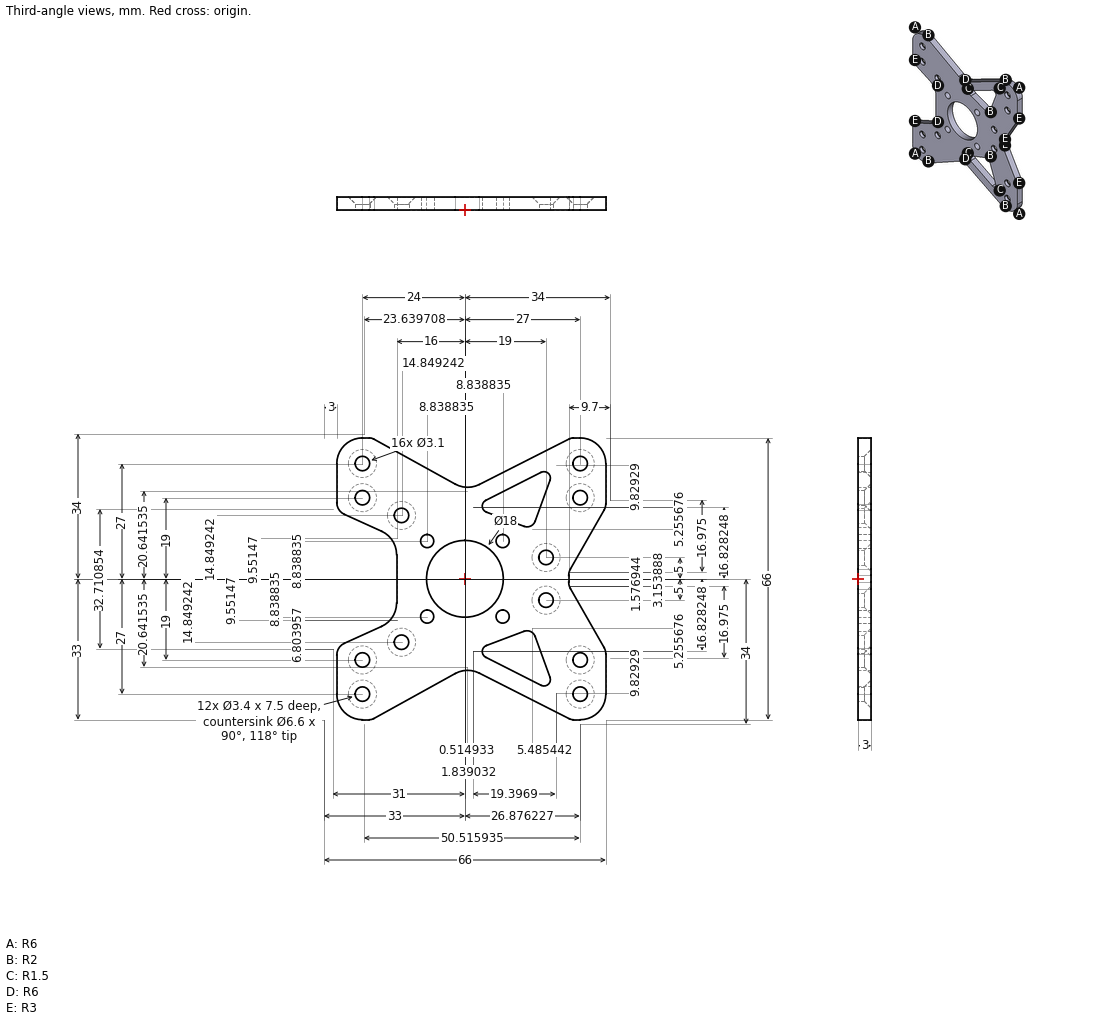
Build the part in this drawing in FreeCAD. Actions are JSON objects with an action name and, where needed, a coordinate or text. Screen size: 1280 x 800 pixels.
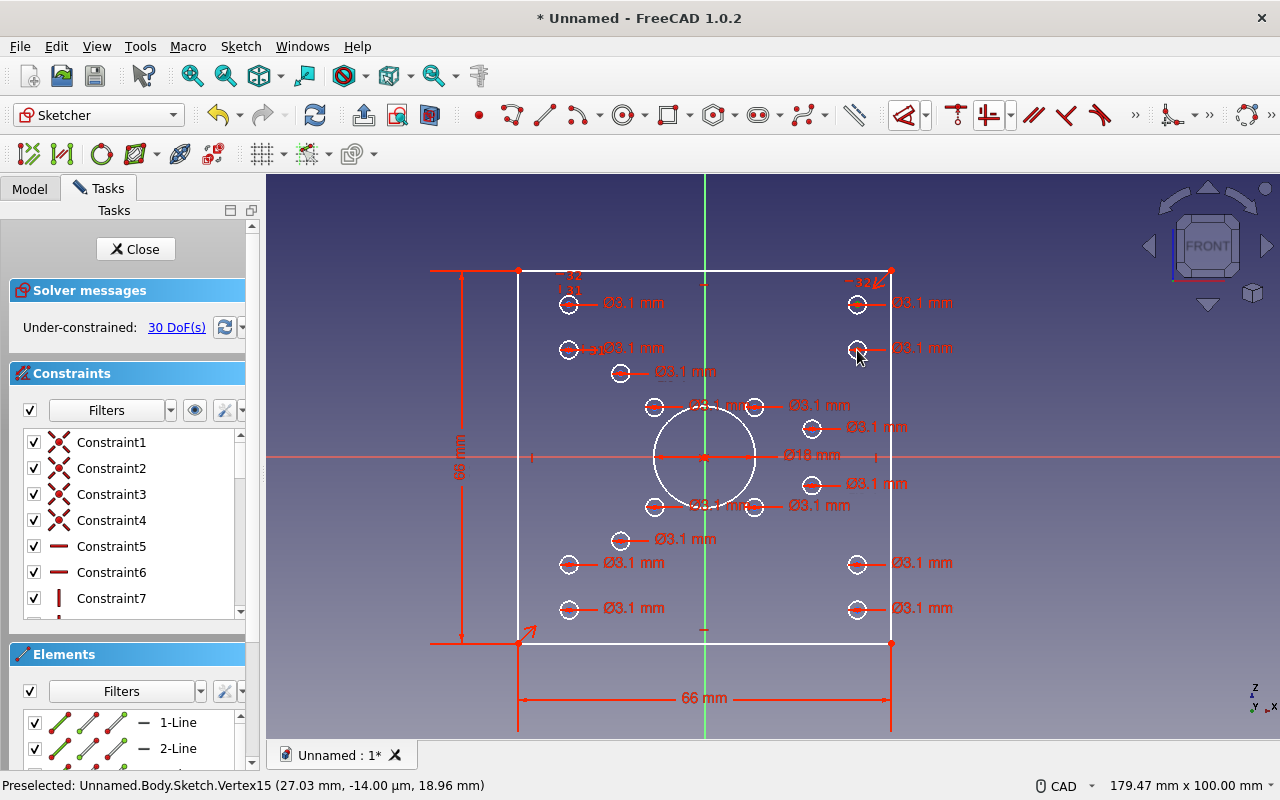
{"action": "key", "text": "v"}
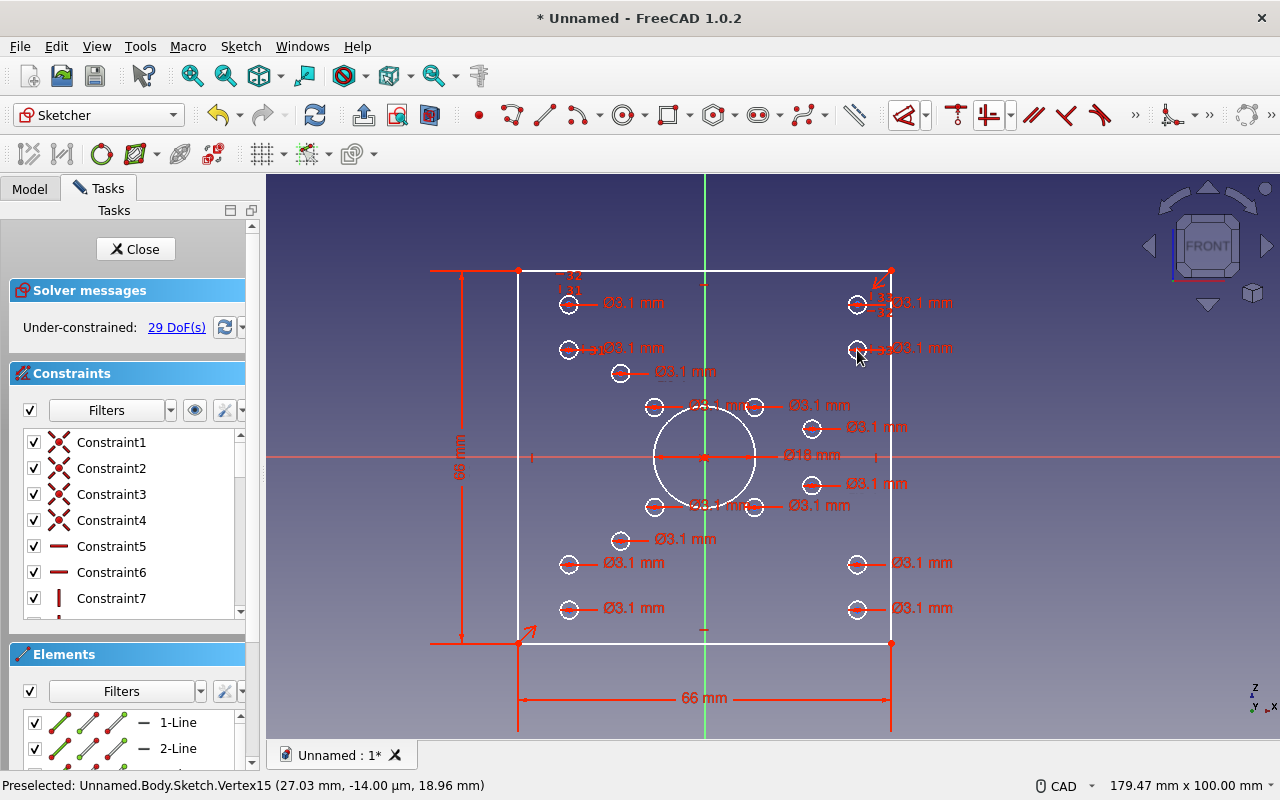
{"action": "left_click", "coordinate": [569, 350]}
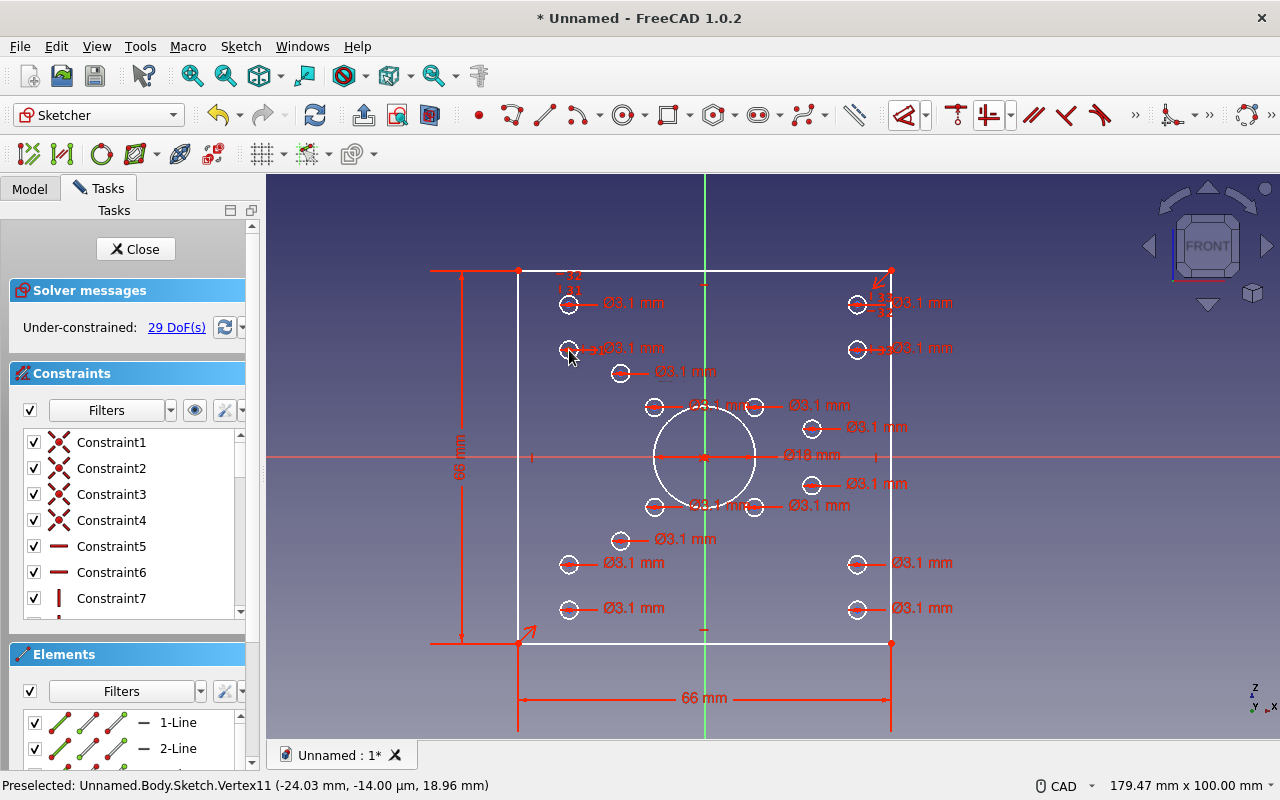
{"action": "left_click", "coordinate": [857, 350]}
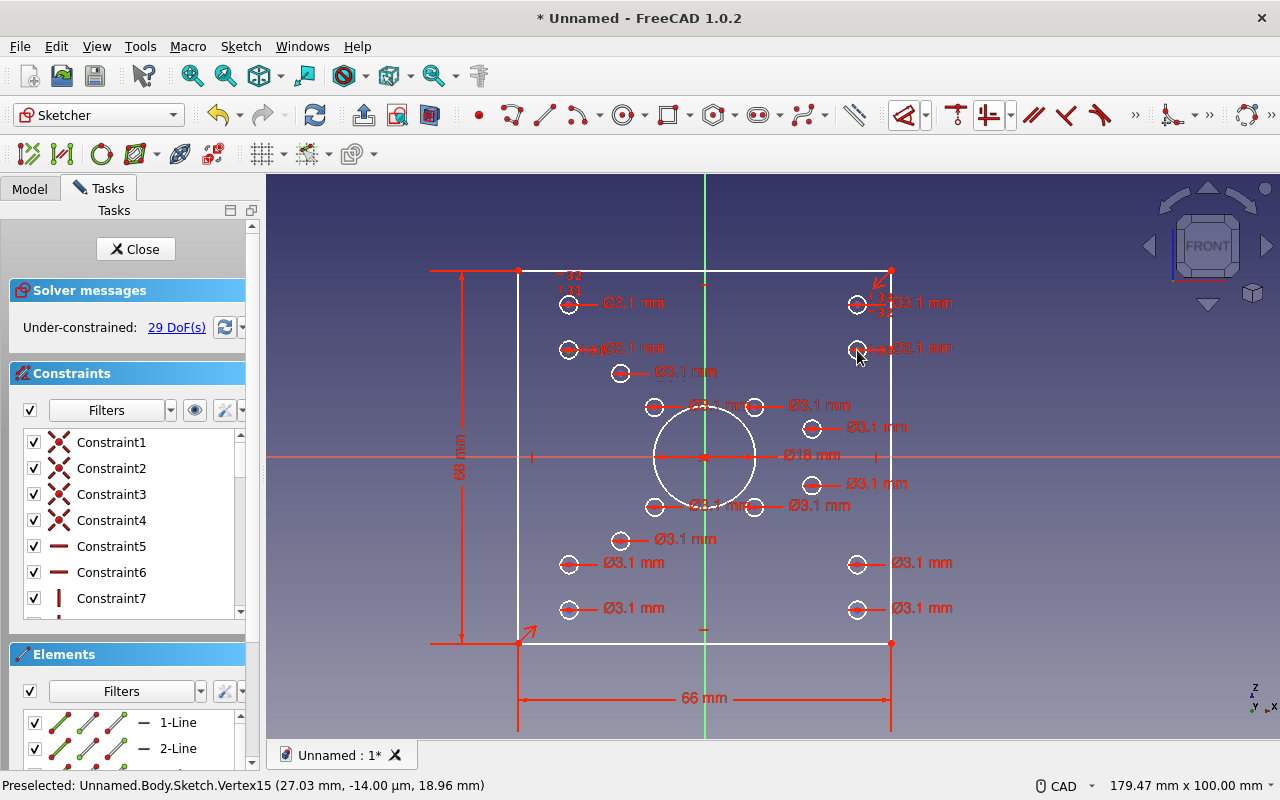
{"action": "key", "text": "h"}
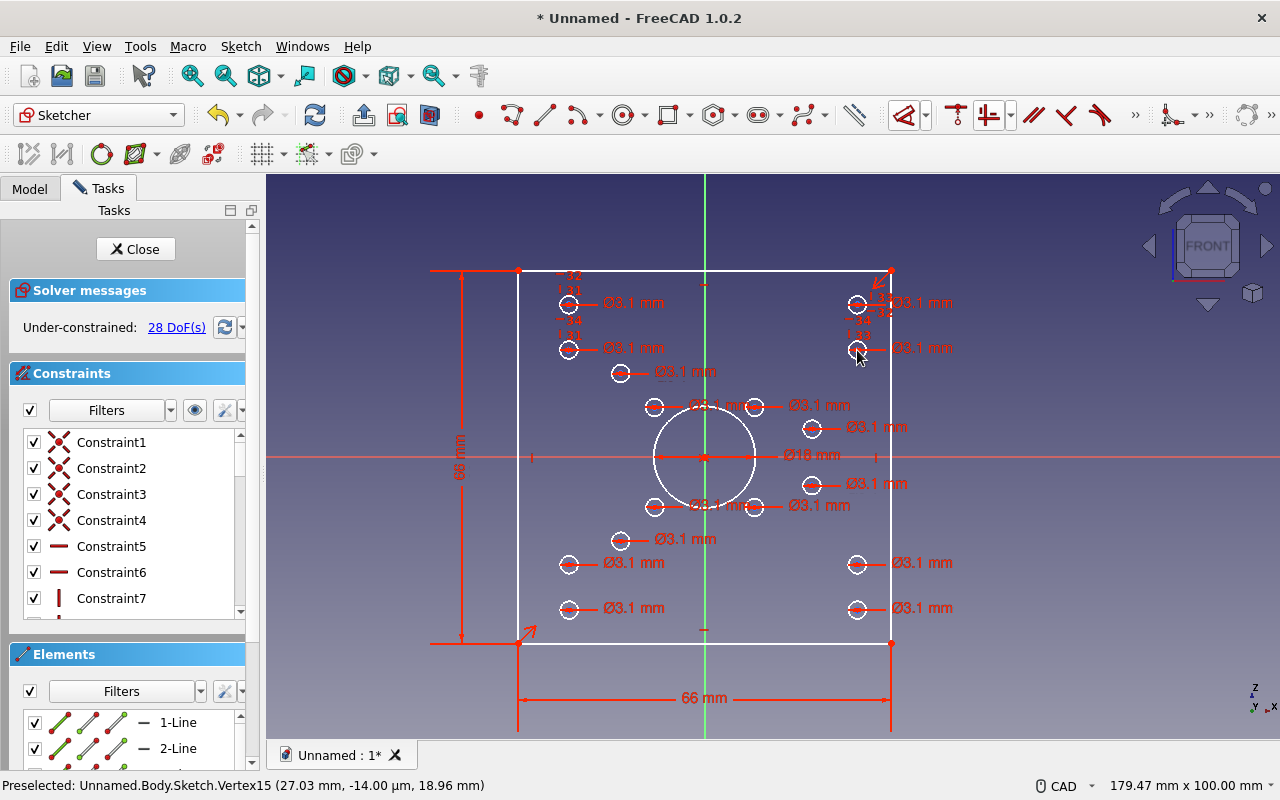
{"action": "left_click", "coordinate": [655, 407]}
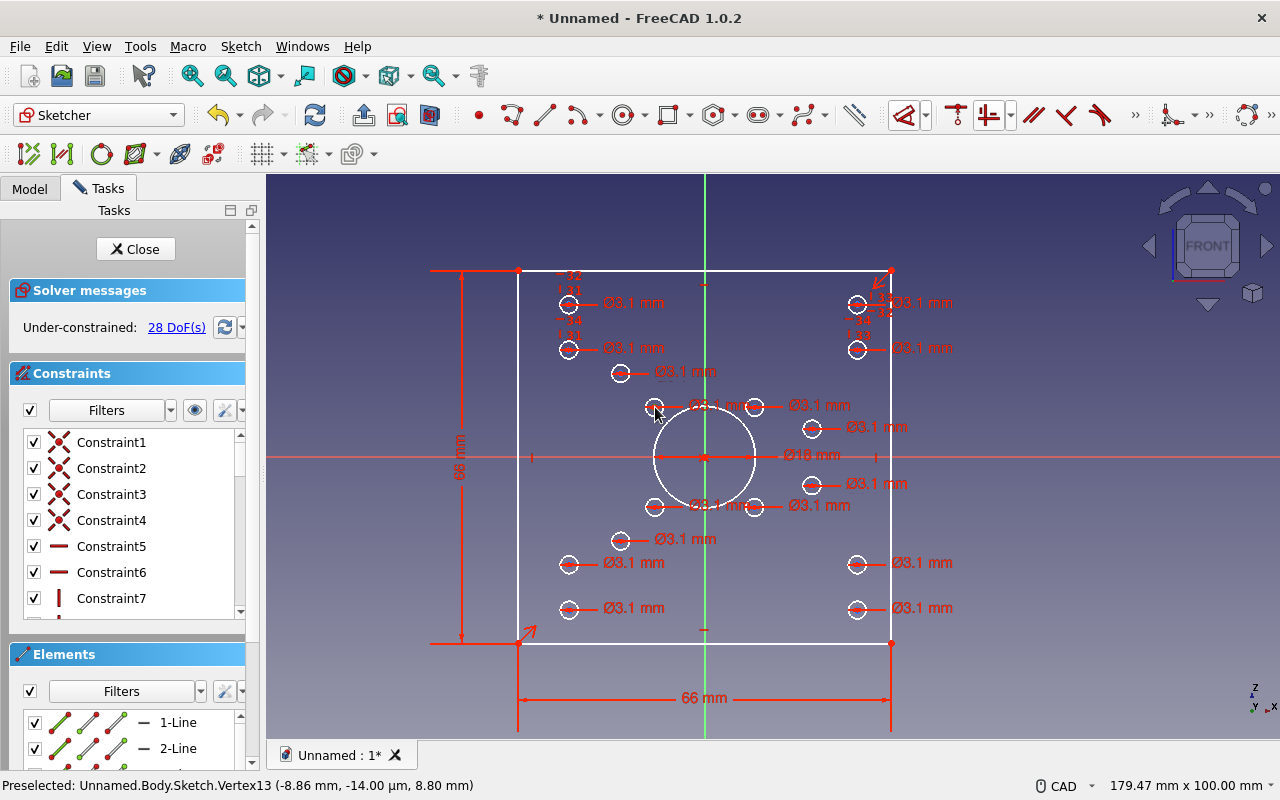
{"action": "left_click", "coordinate": [755, 407]}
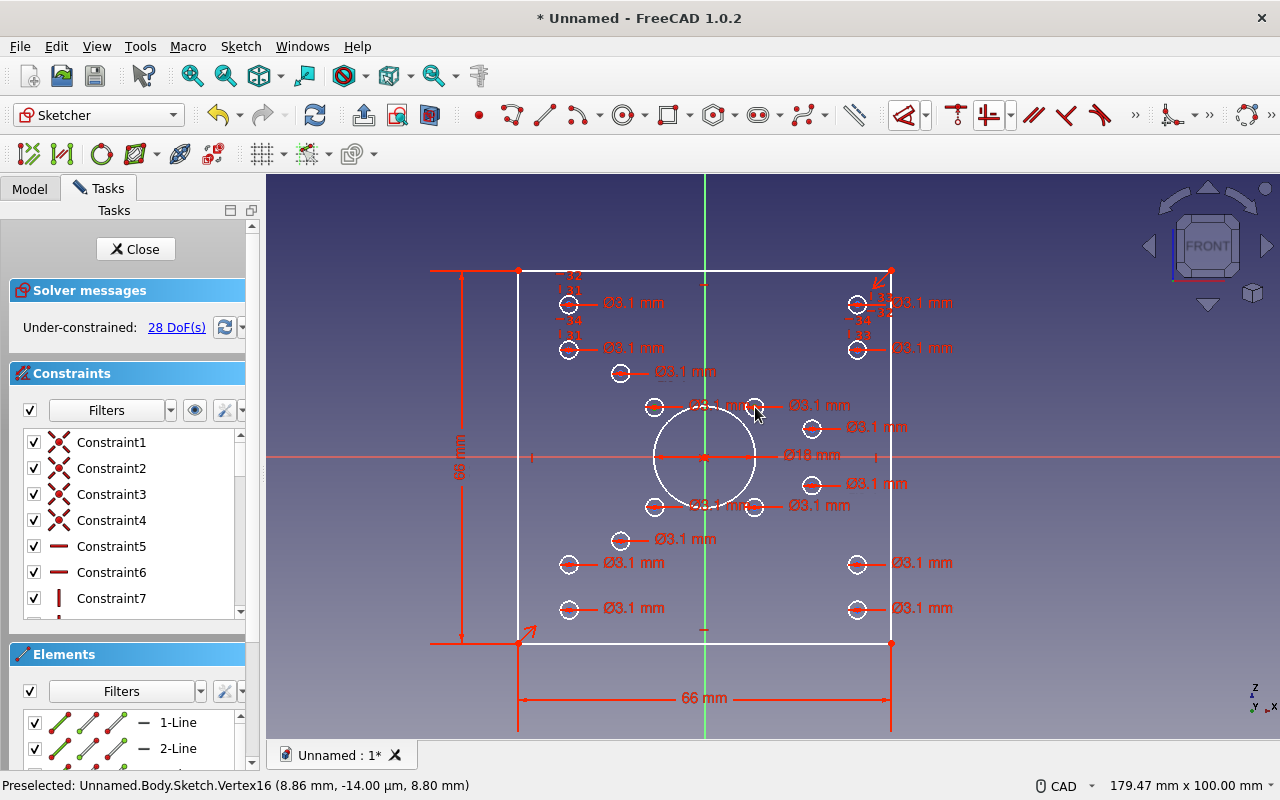
{"action": "left_click", "coordinate": [1010, 116]}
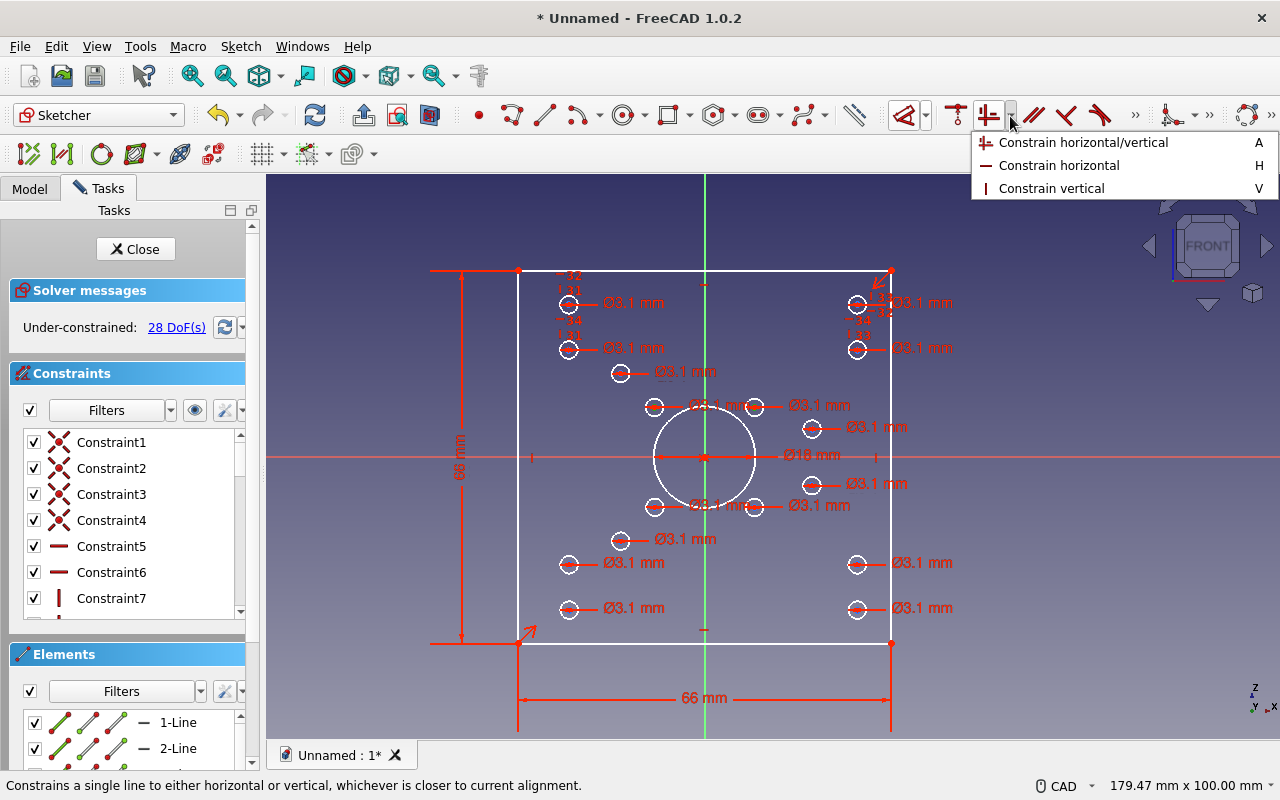
{"action": "left_click", "coordinate": [1125, 166]}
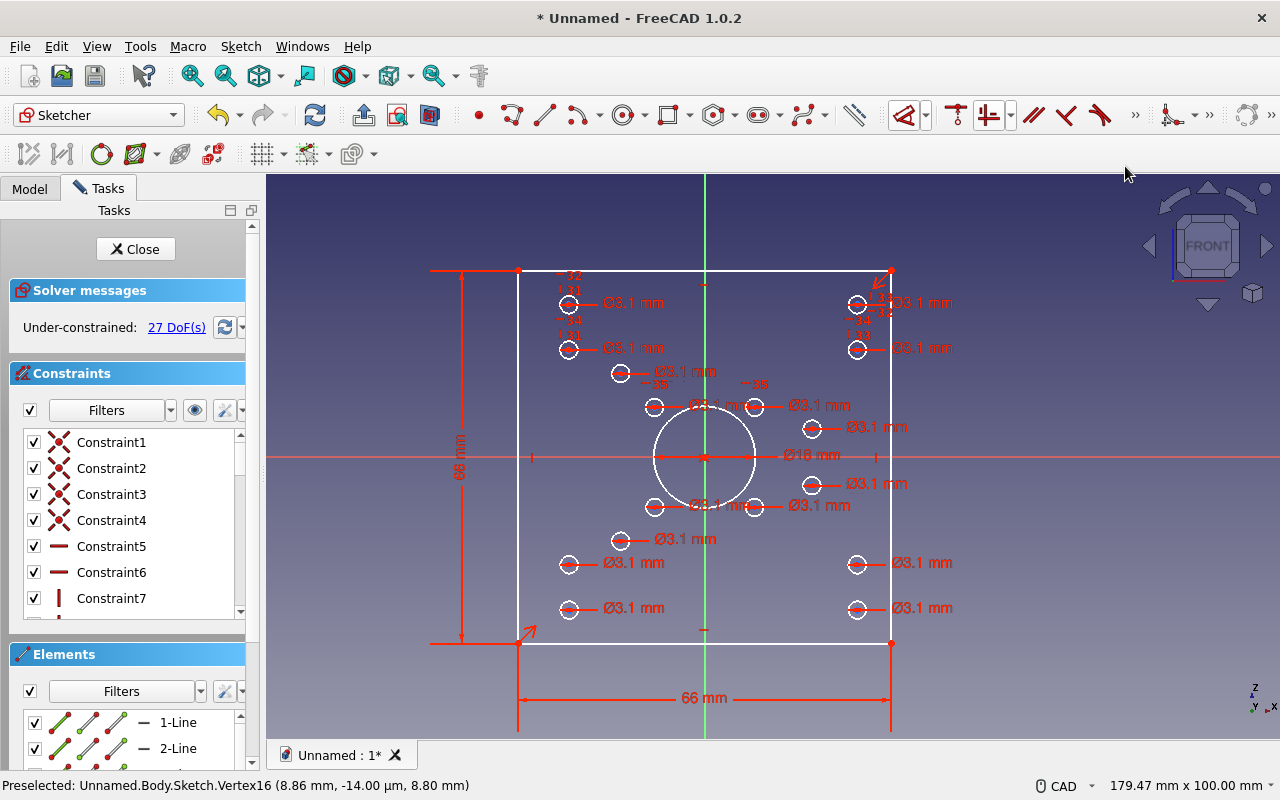
{"action": "left_click", "coordinate": [655, 407]}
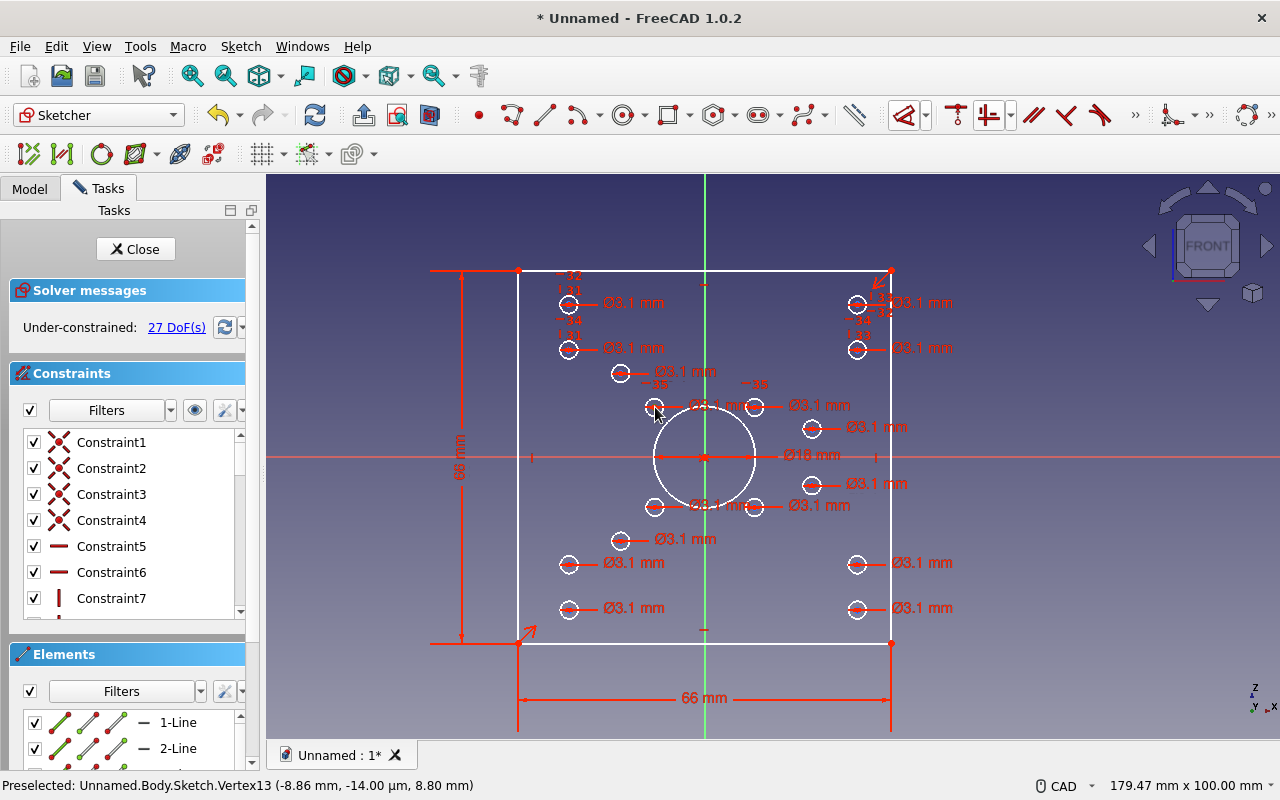
{"action": "left_click", "coordinate": [655, 507]}